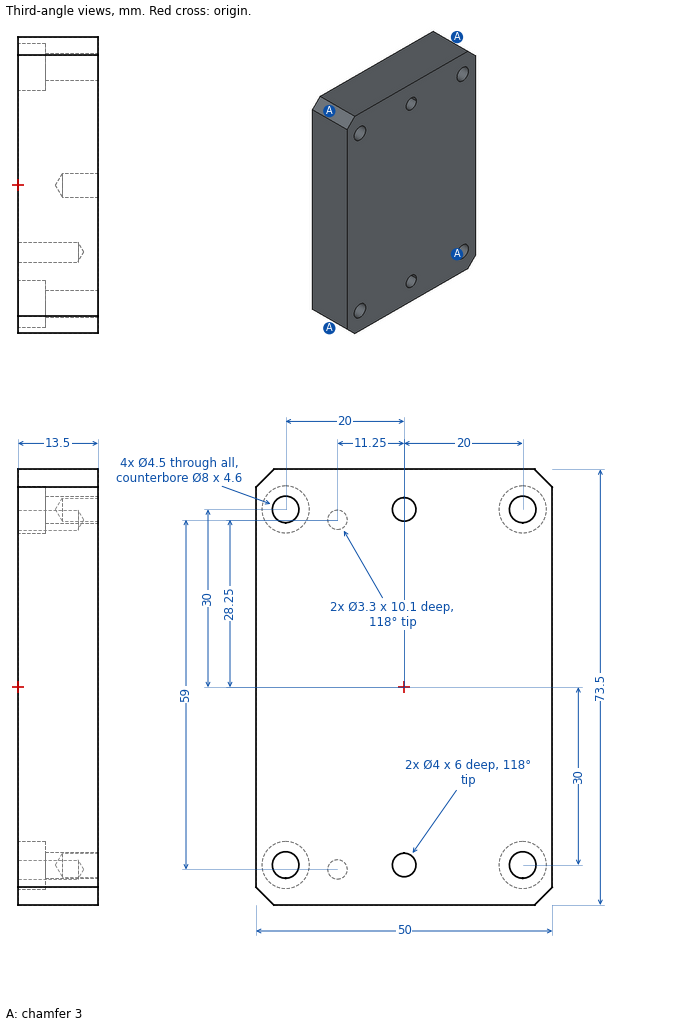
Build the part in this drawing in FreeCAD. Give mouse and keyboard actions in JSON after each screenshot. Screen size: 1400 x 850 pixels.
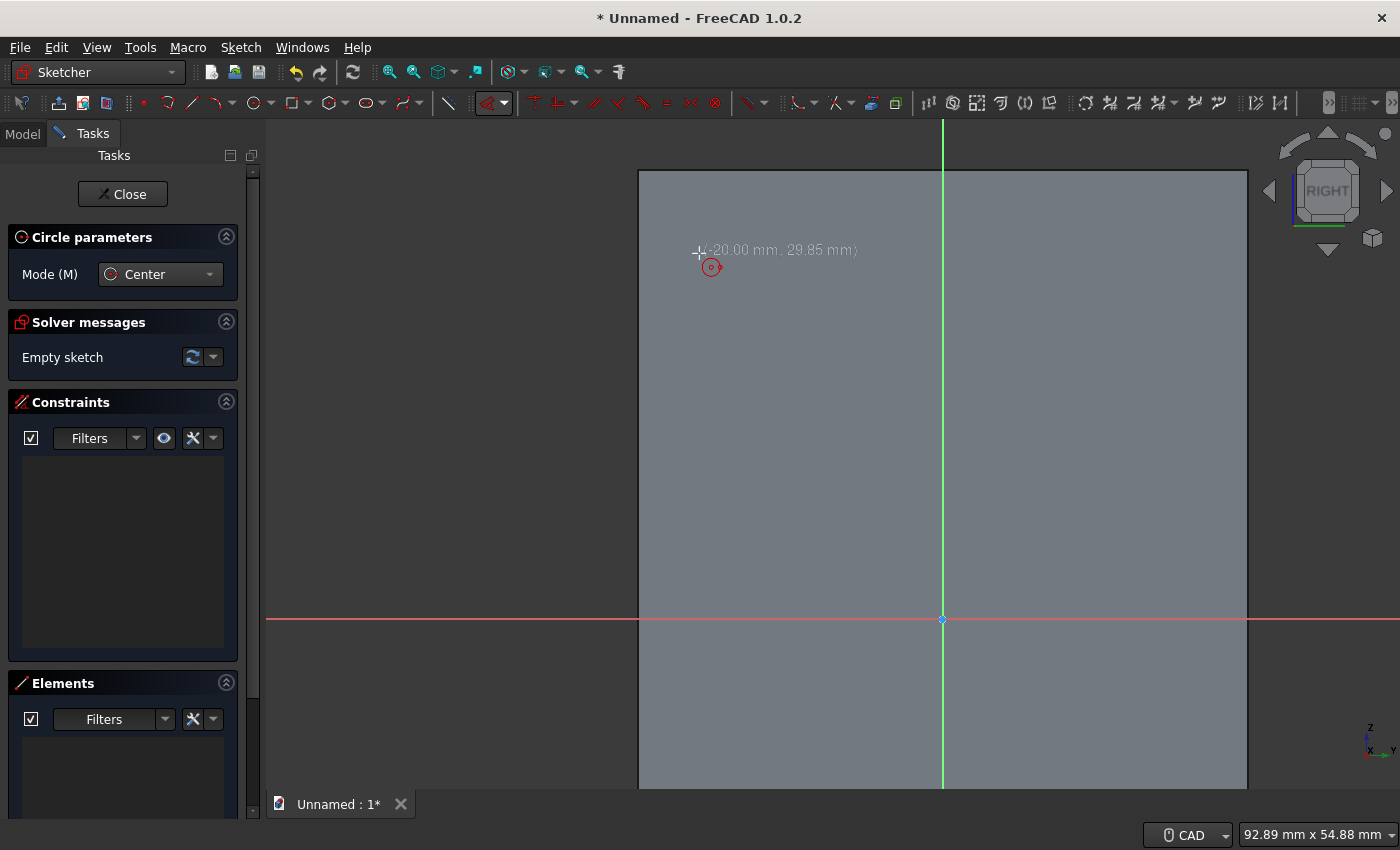
{"action": "left_click", "coordinate": [699, 253]}
{"action": "mouse_move", "coordinate": [718, 233]}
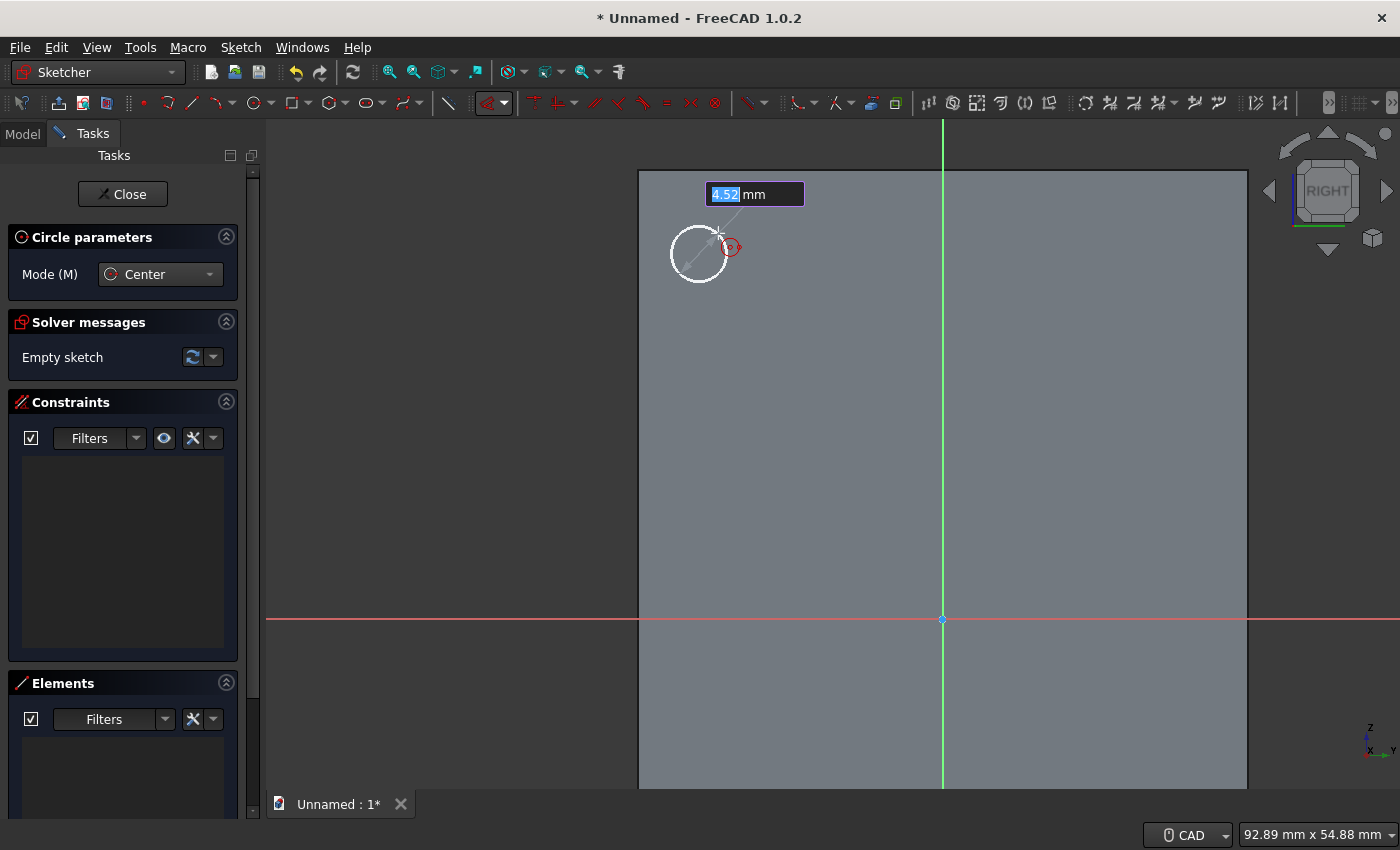
{"action": "type", "text": "4.5"}
{"action": "key", "text": "Return"}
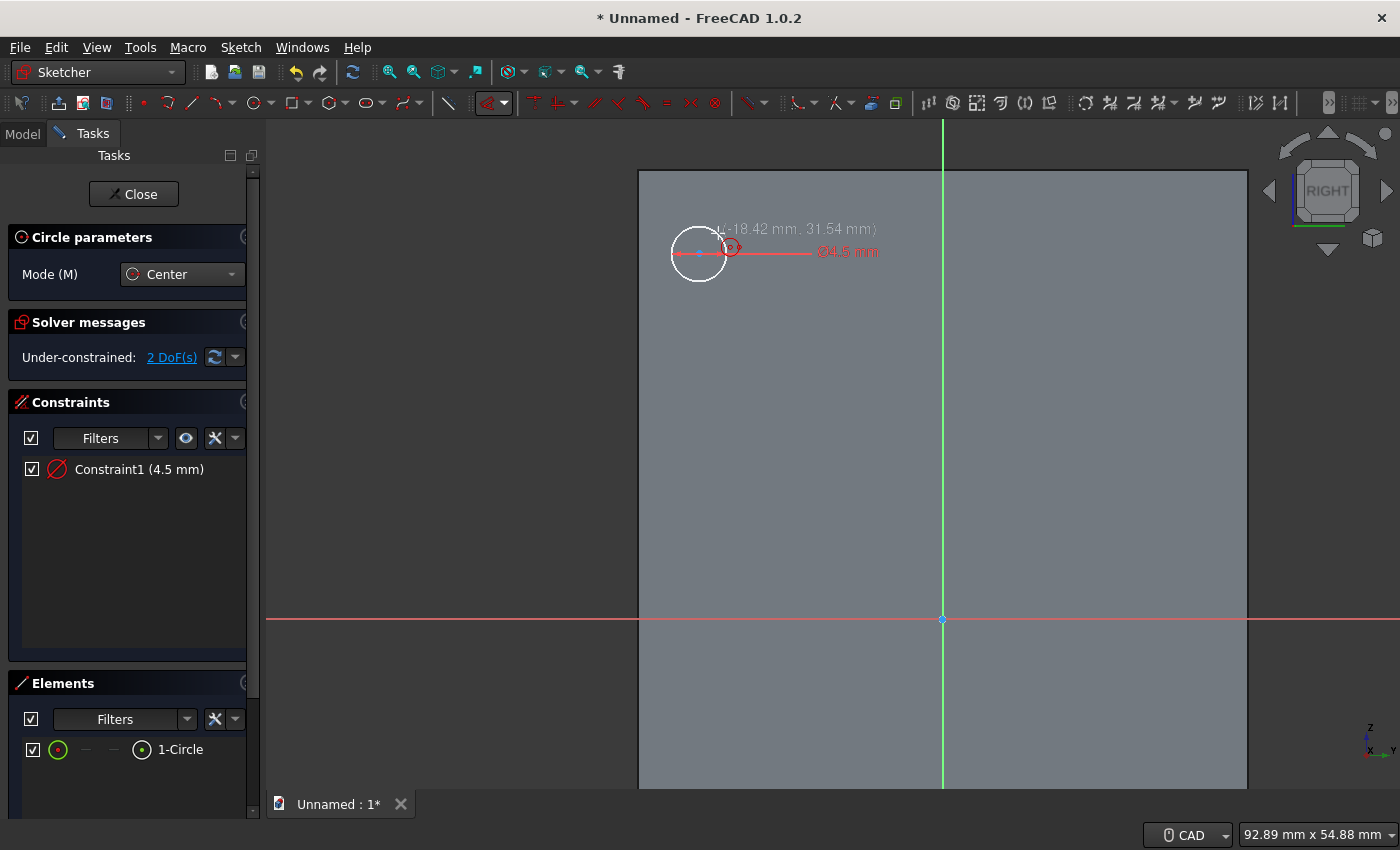
{"action": "left_click", "coordinate": [1187, 253]}
{"action": "mouse_move", "coordinate": [1206, 233]}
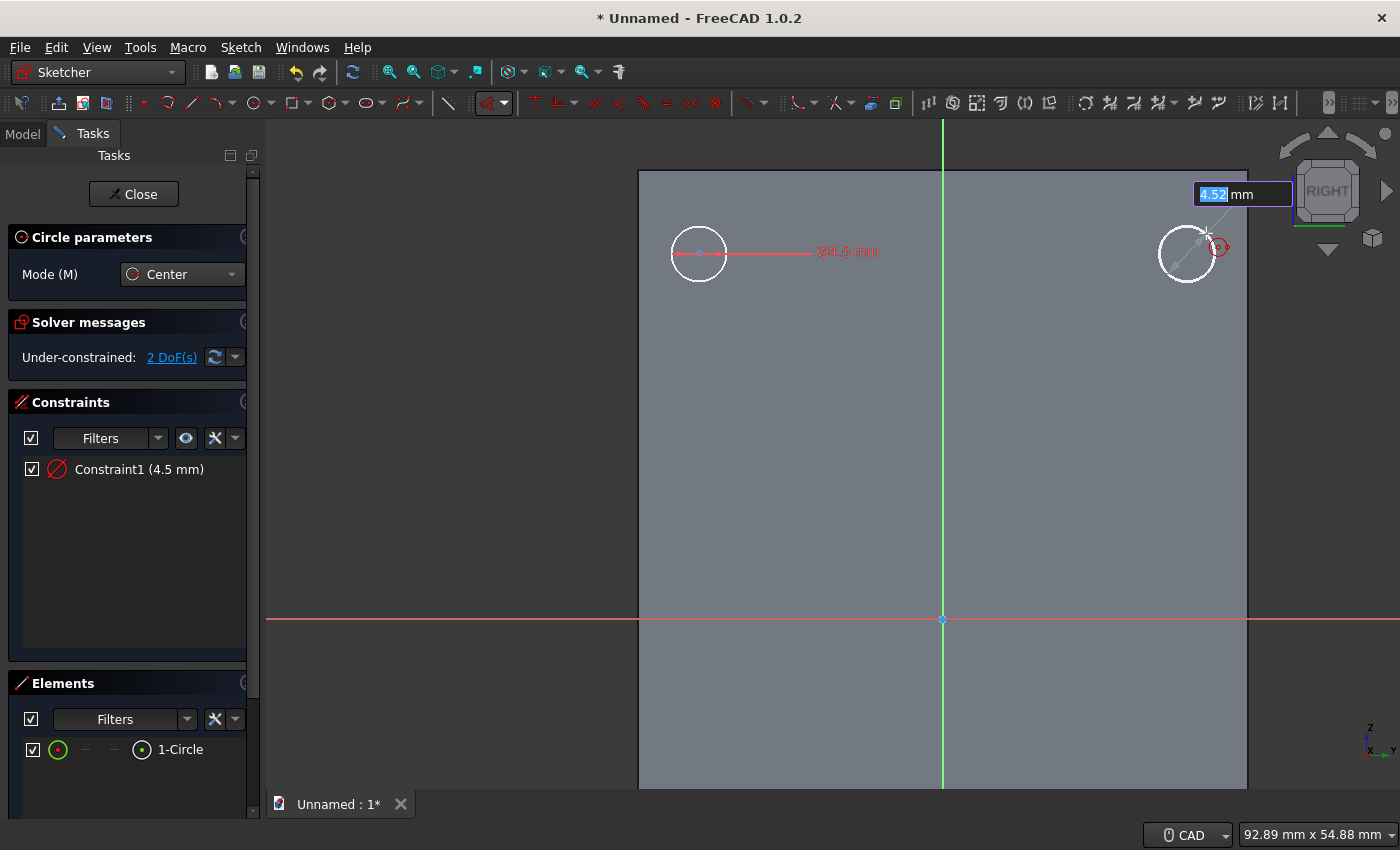
{"action": "type", "text": "4.5"}
{"action": "key", "text": "Return"}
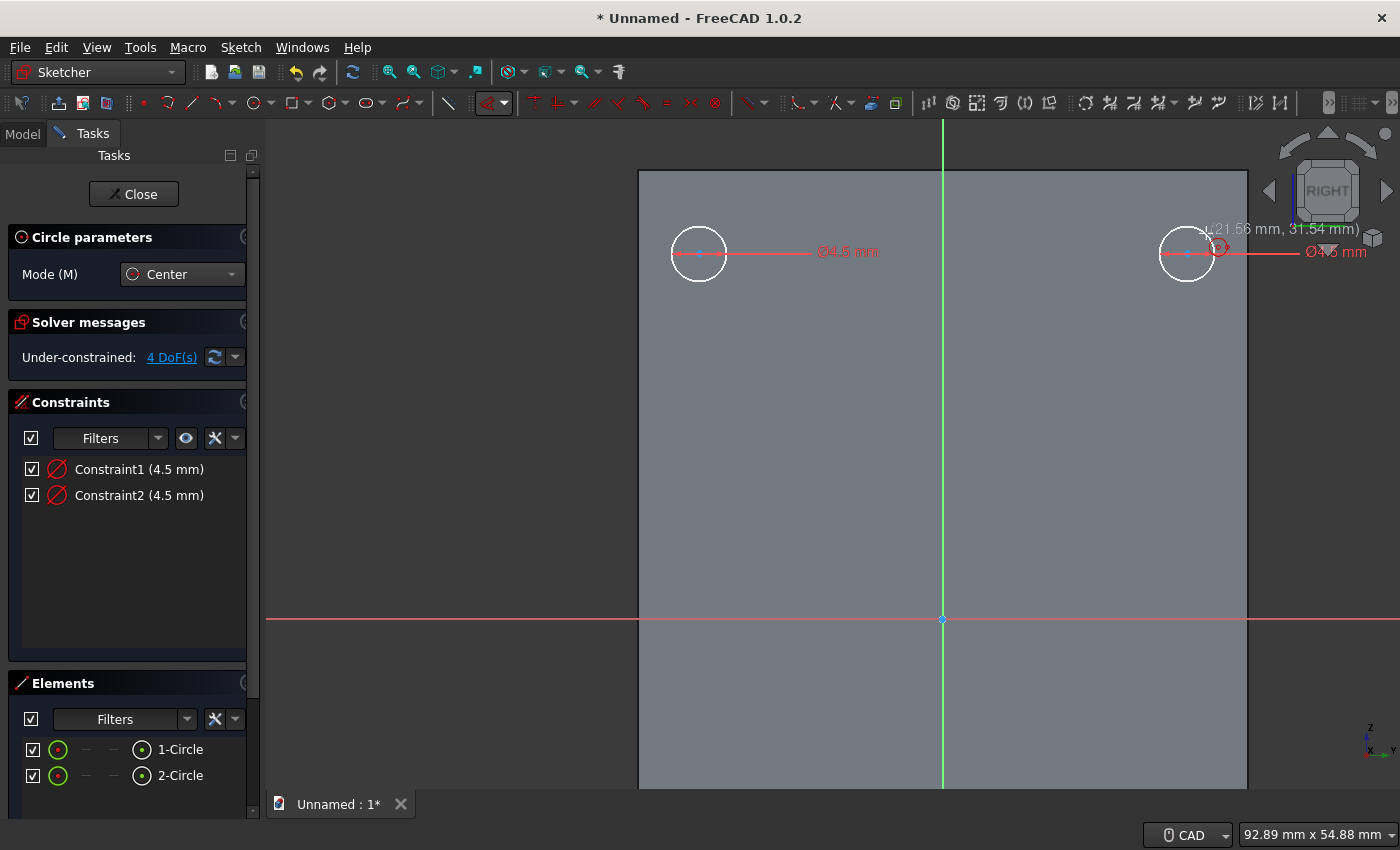
{"action": "scroll", "coordinate": [548, 253], "scroll_direction": "down", "scroll_amount": 3}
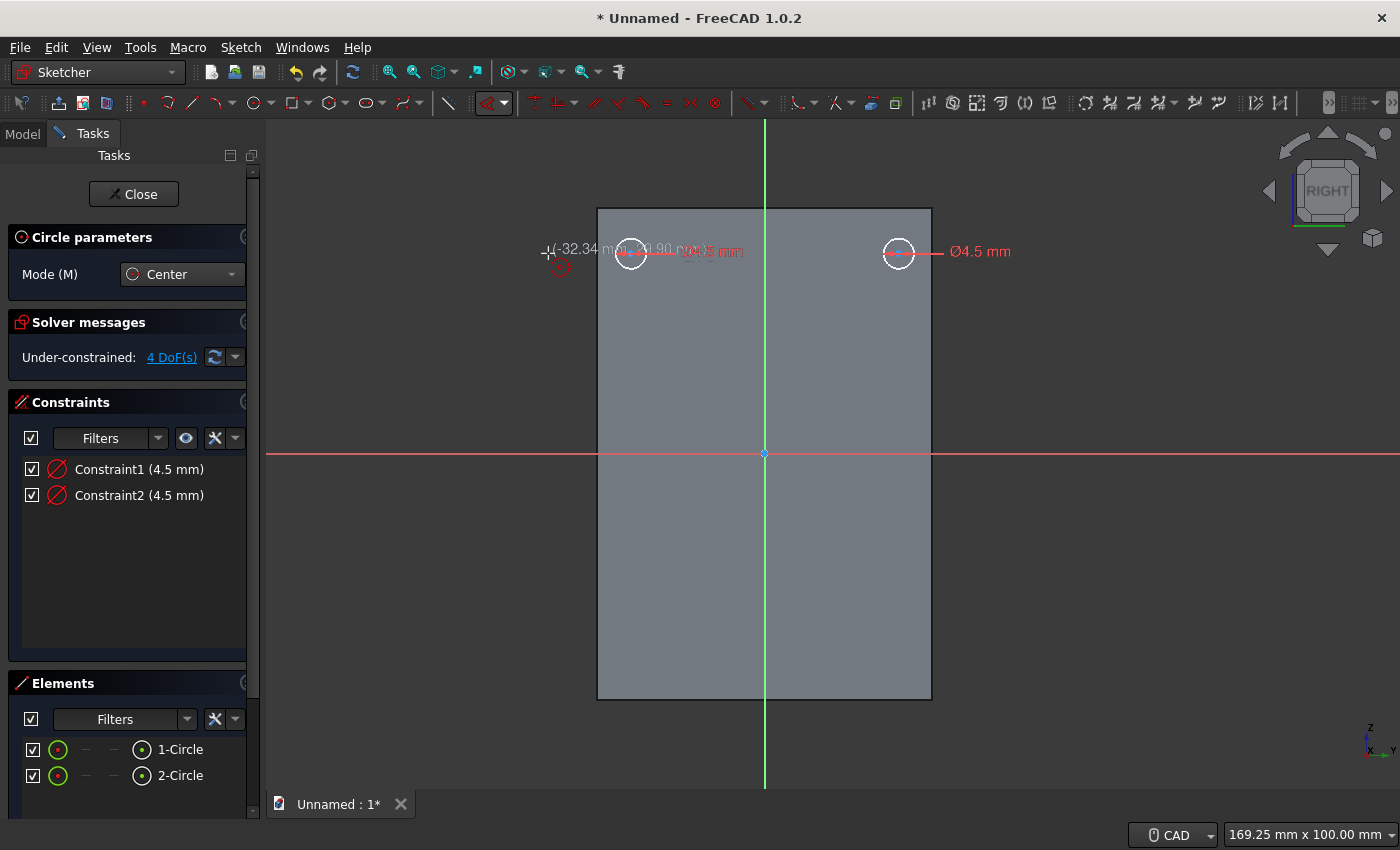
{"action": "scroll", "coordinate": [899, 655], "scroll_direction": "up", "scroll_amount": 3}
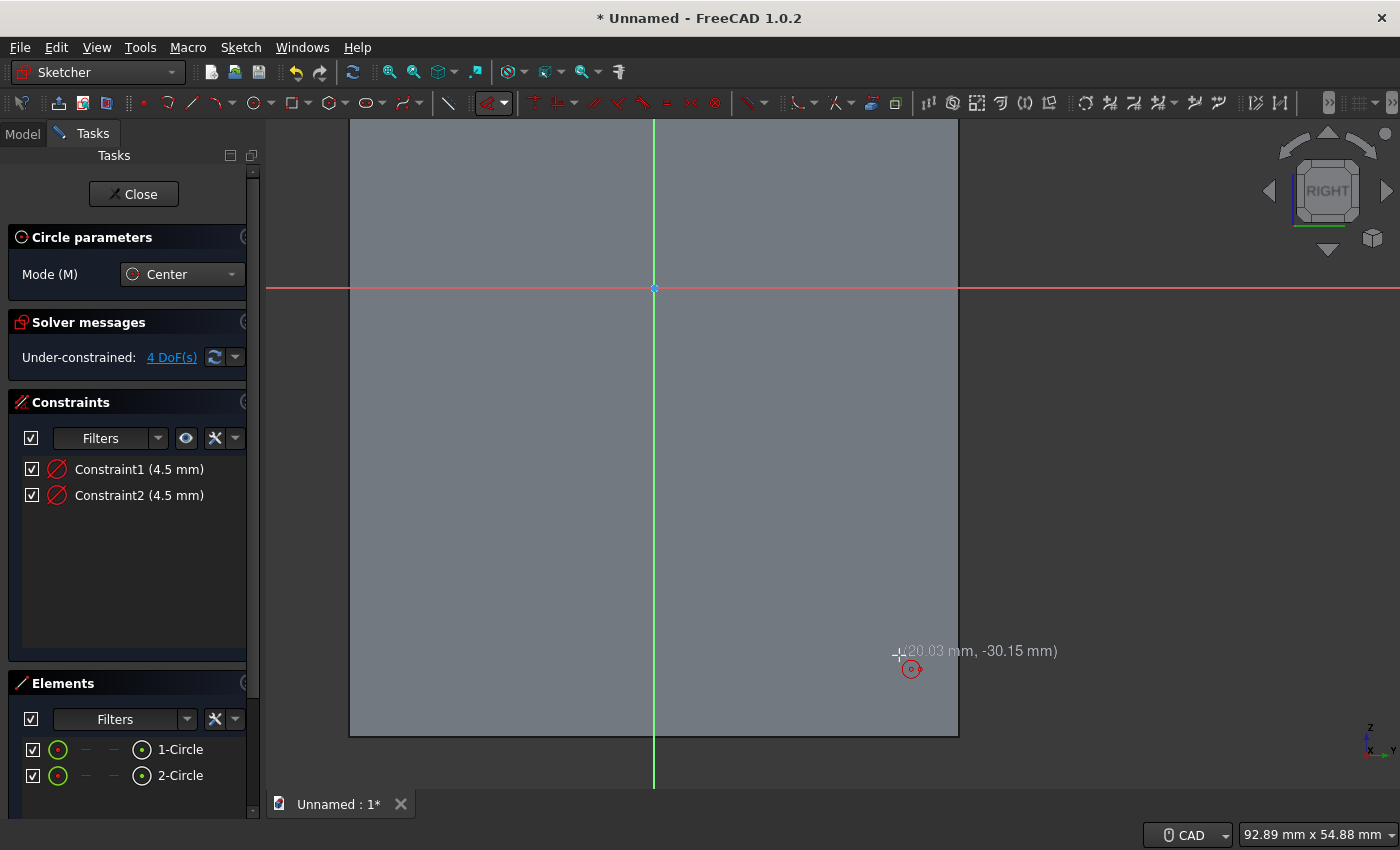
{"action": "left_click", "coordinate": [898, 654]}
{"action": "mouse_move", "coordinate": [918, 635]}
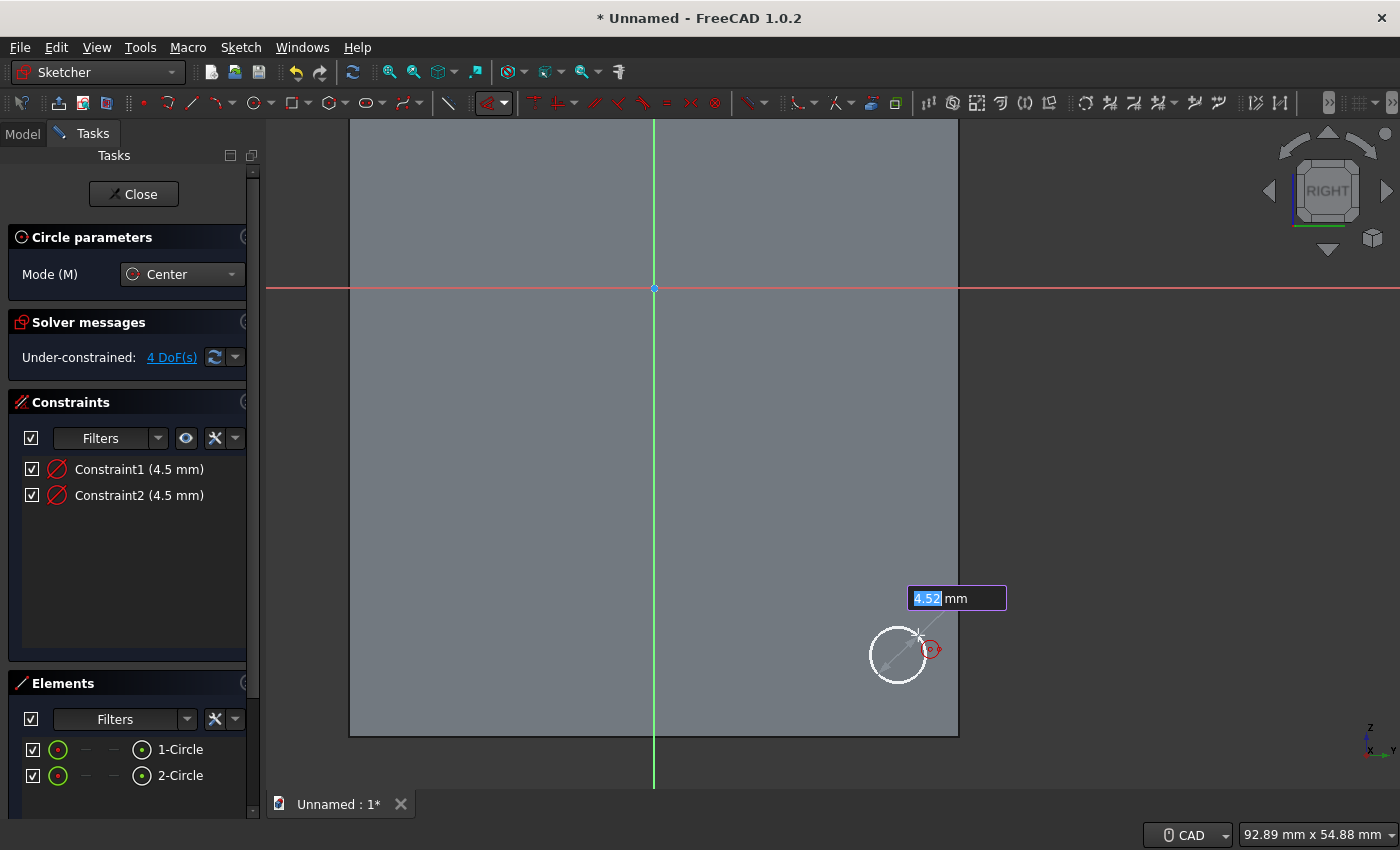
{"action": "type", "text": "4.5"}
{"action": "key", "text": "Return"}